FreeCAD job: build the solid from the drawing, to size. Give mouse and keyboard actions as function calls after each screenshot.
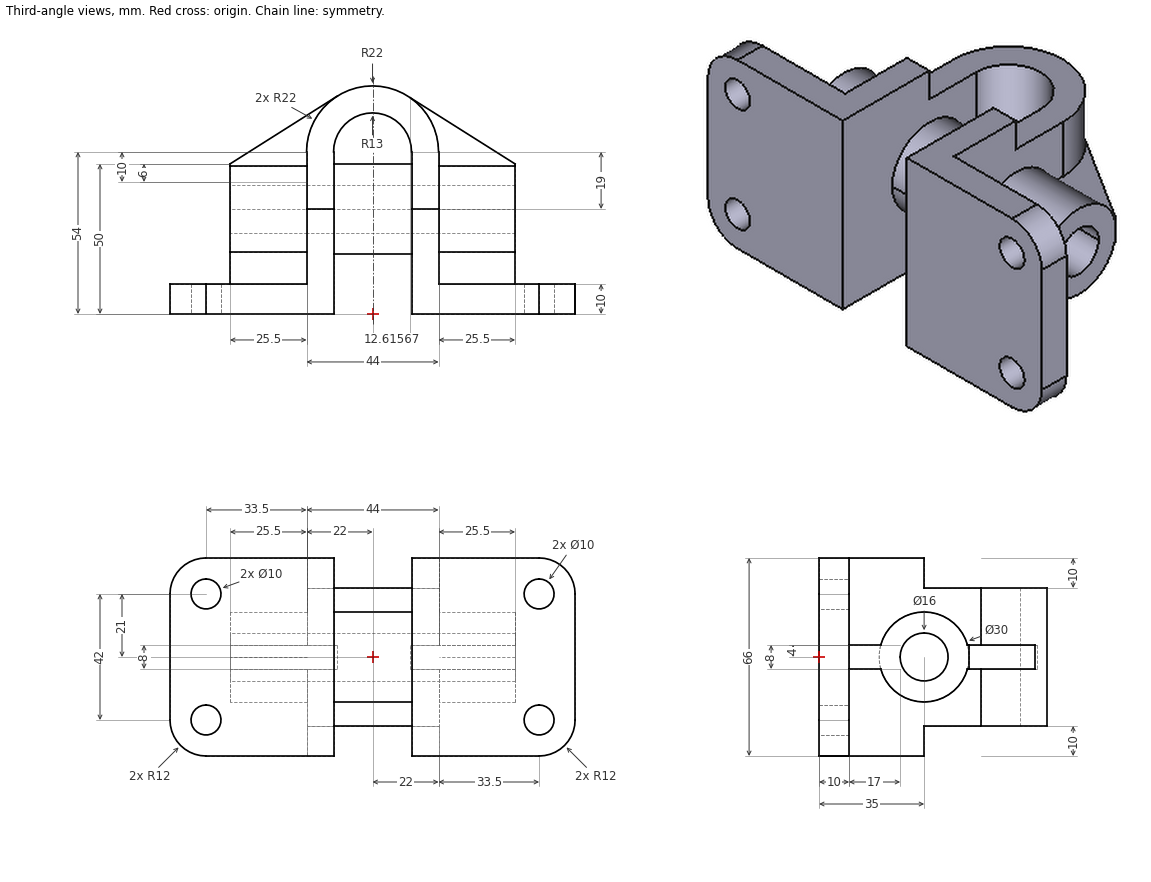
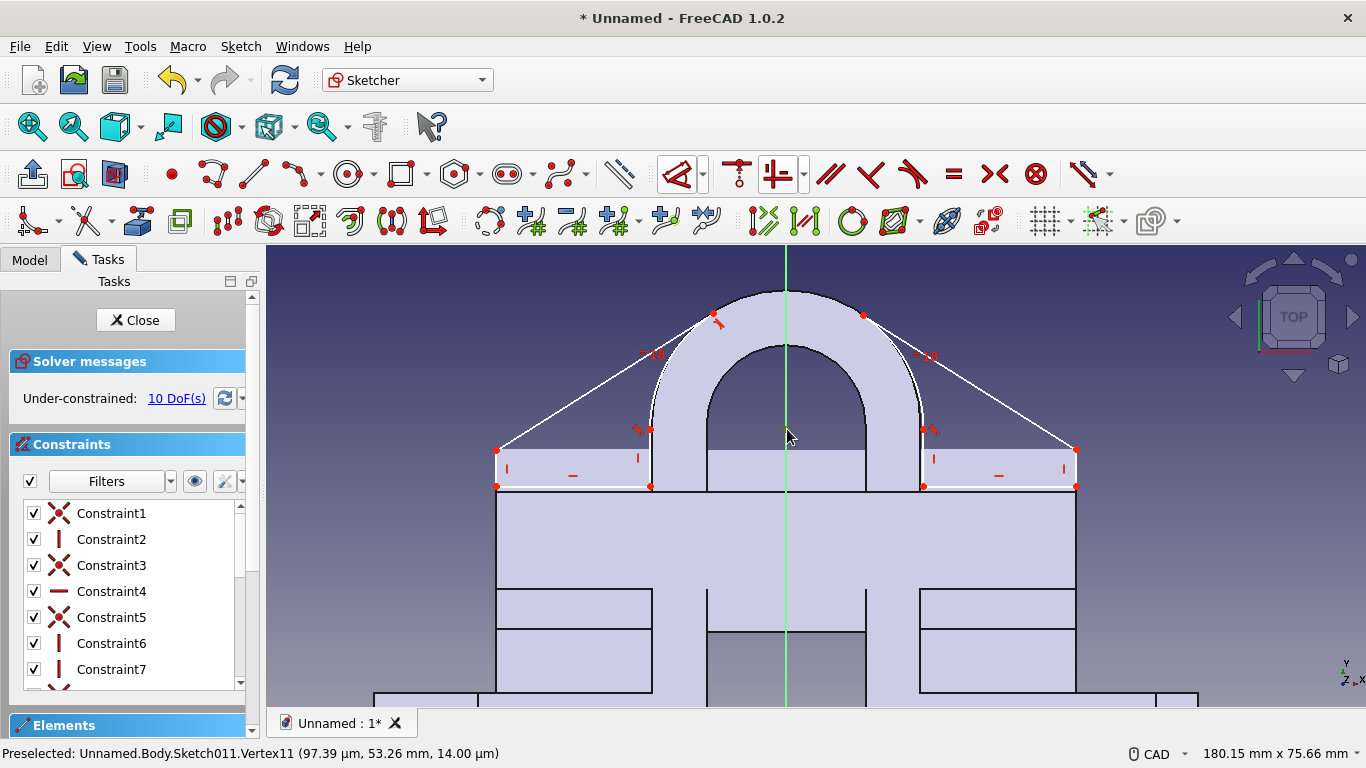
click(786, 650)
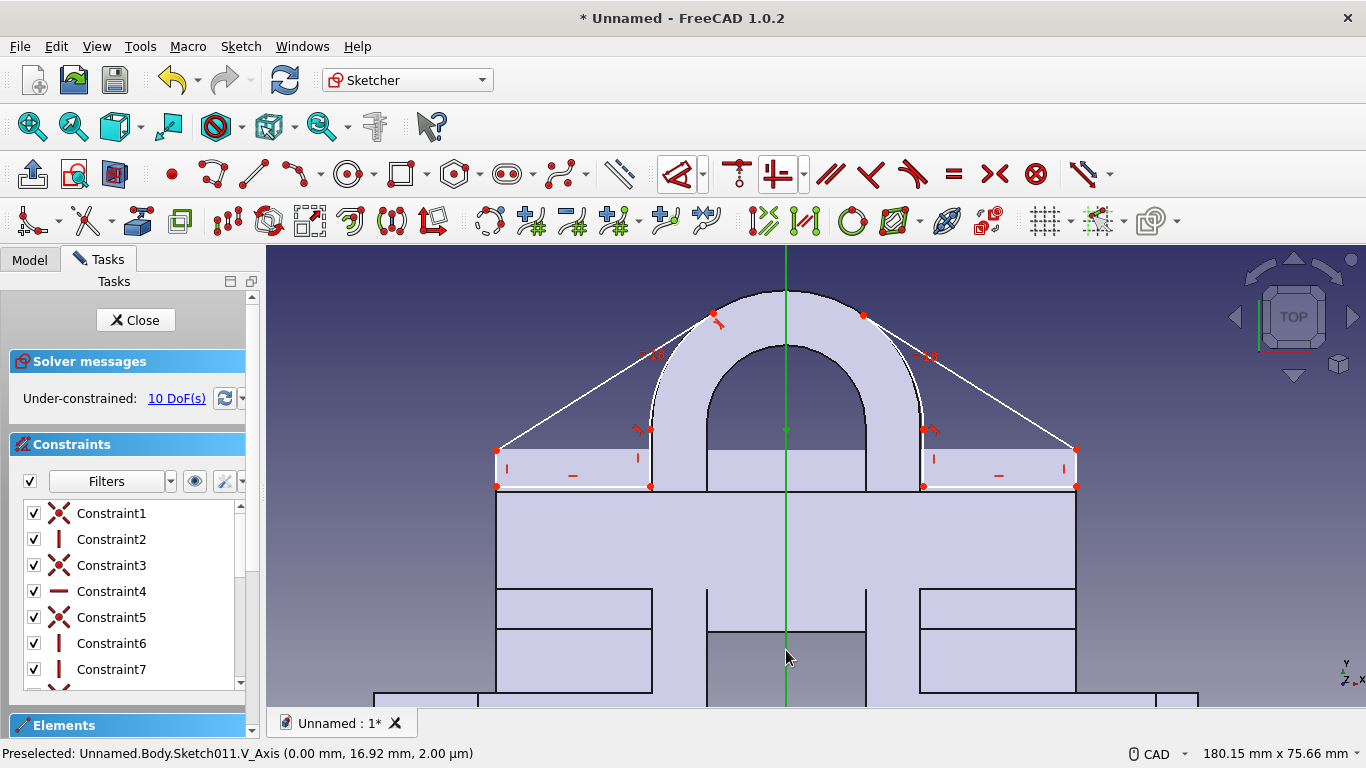
click(737, 174)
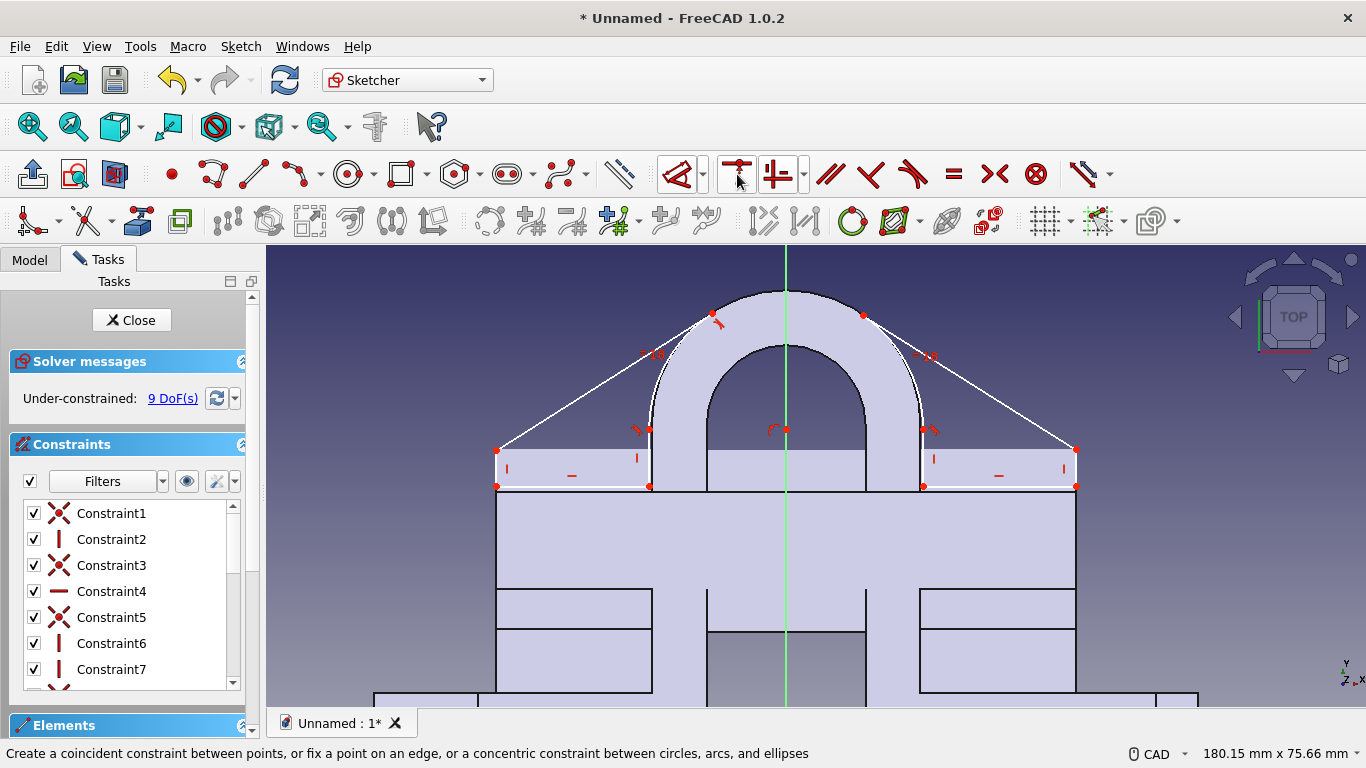
click(496, 487)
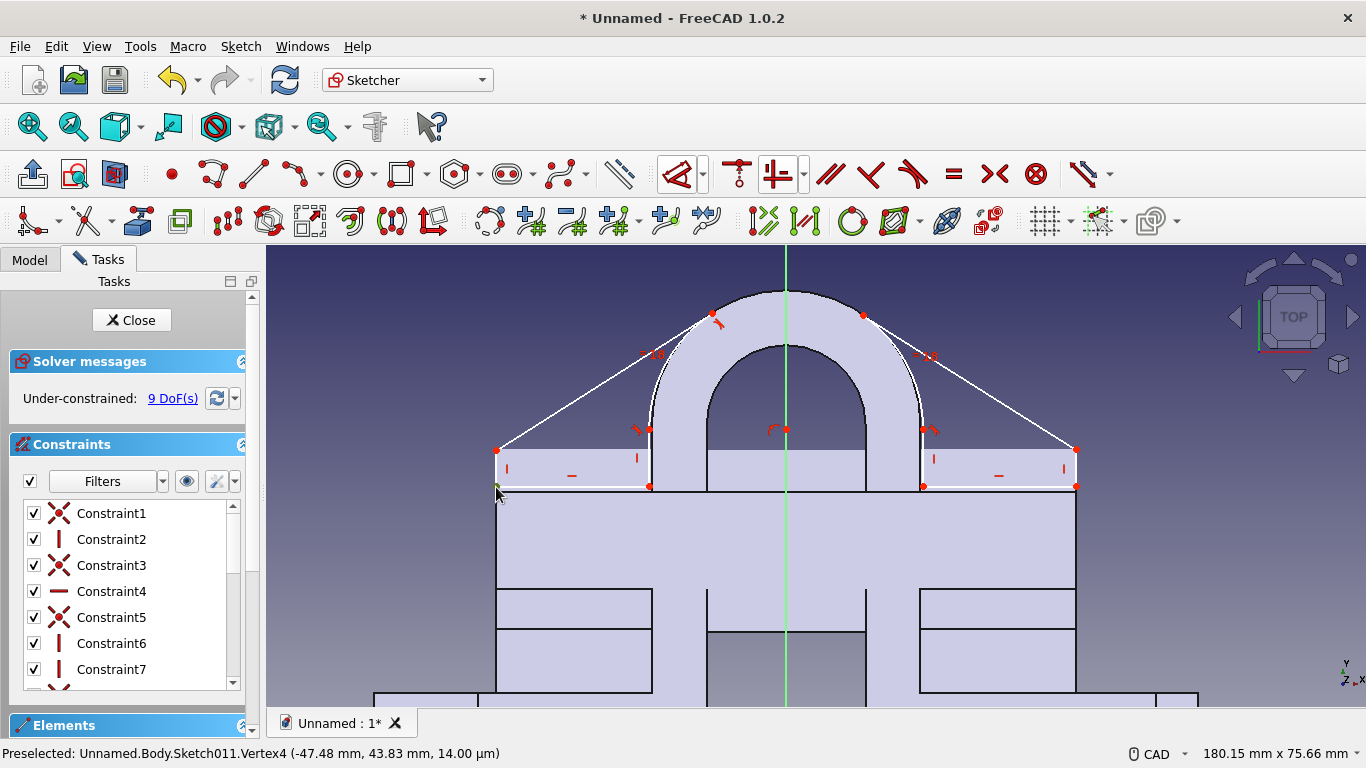
click(1076, 487)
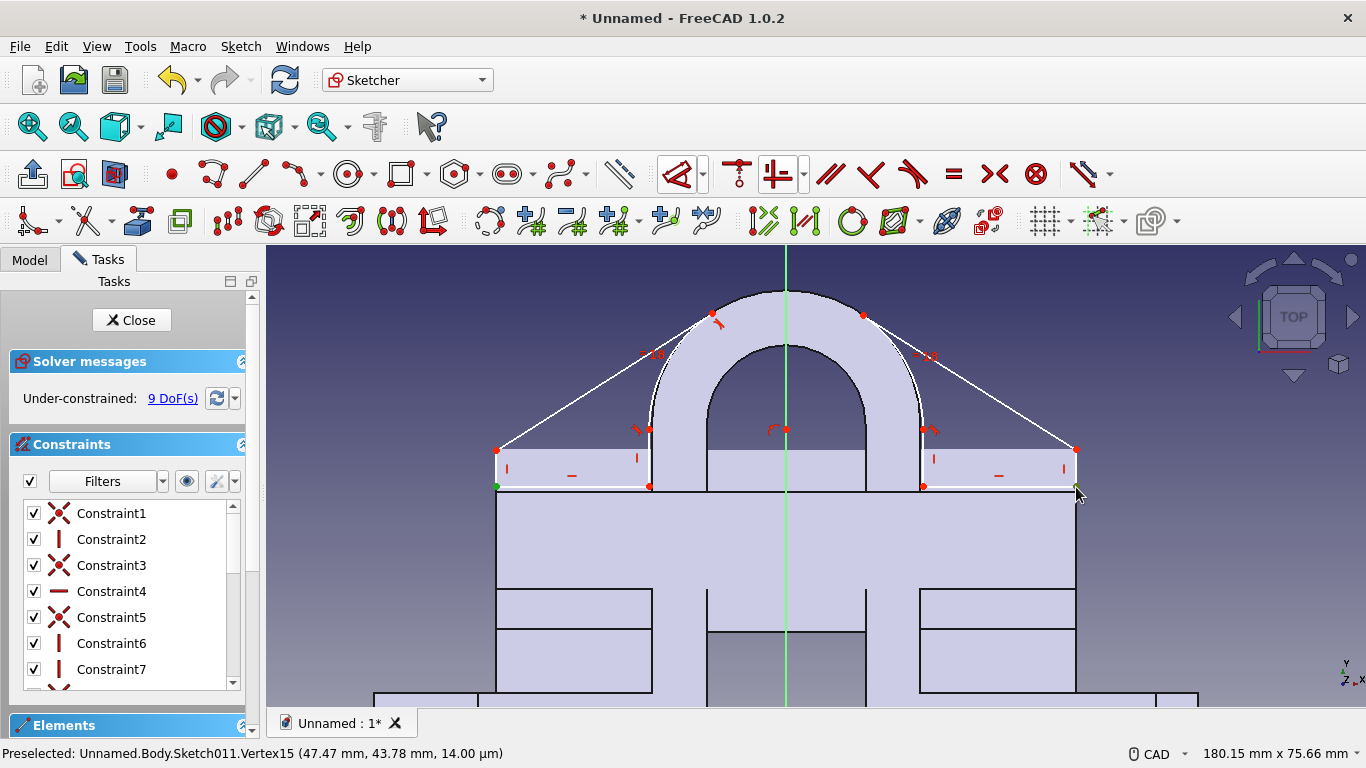
click(786, 650)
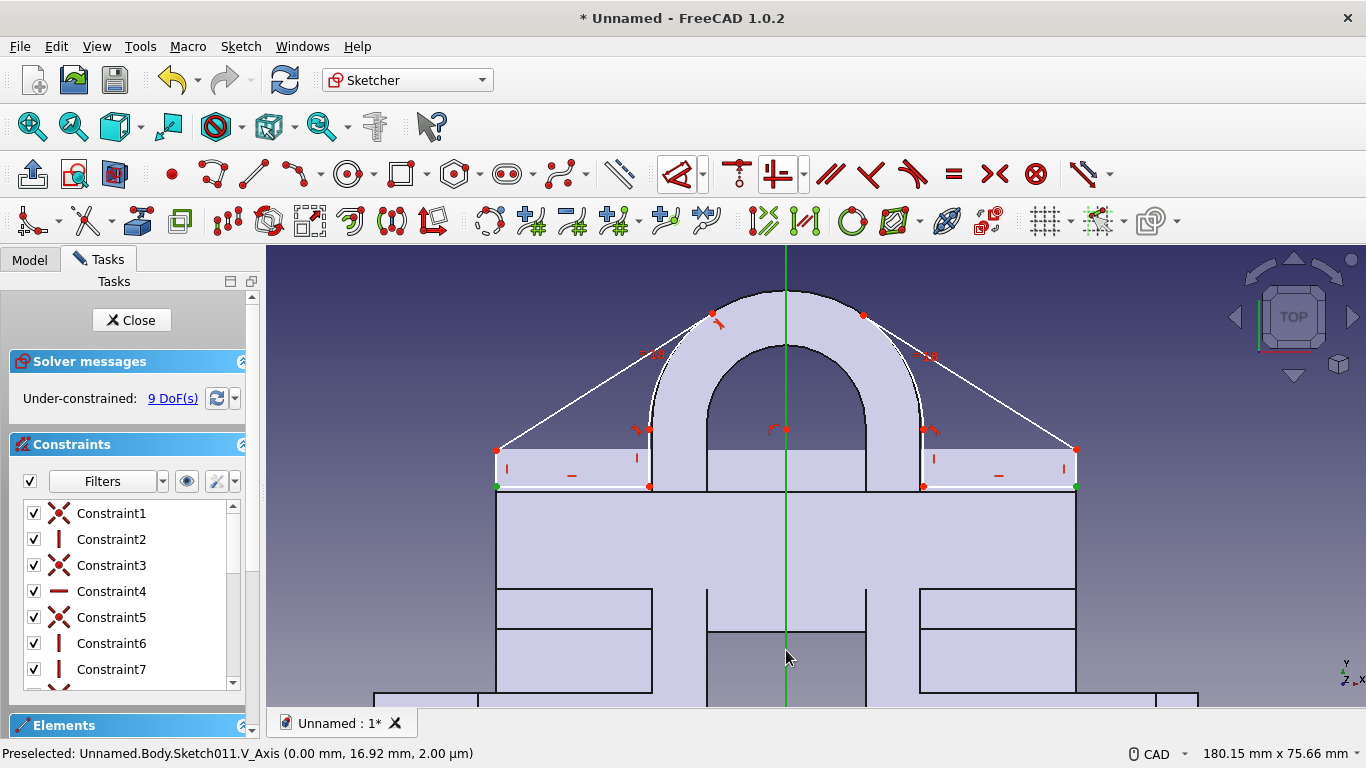
click(995, 174)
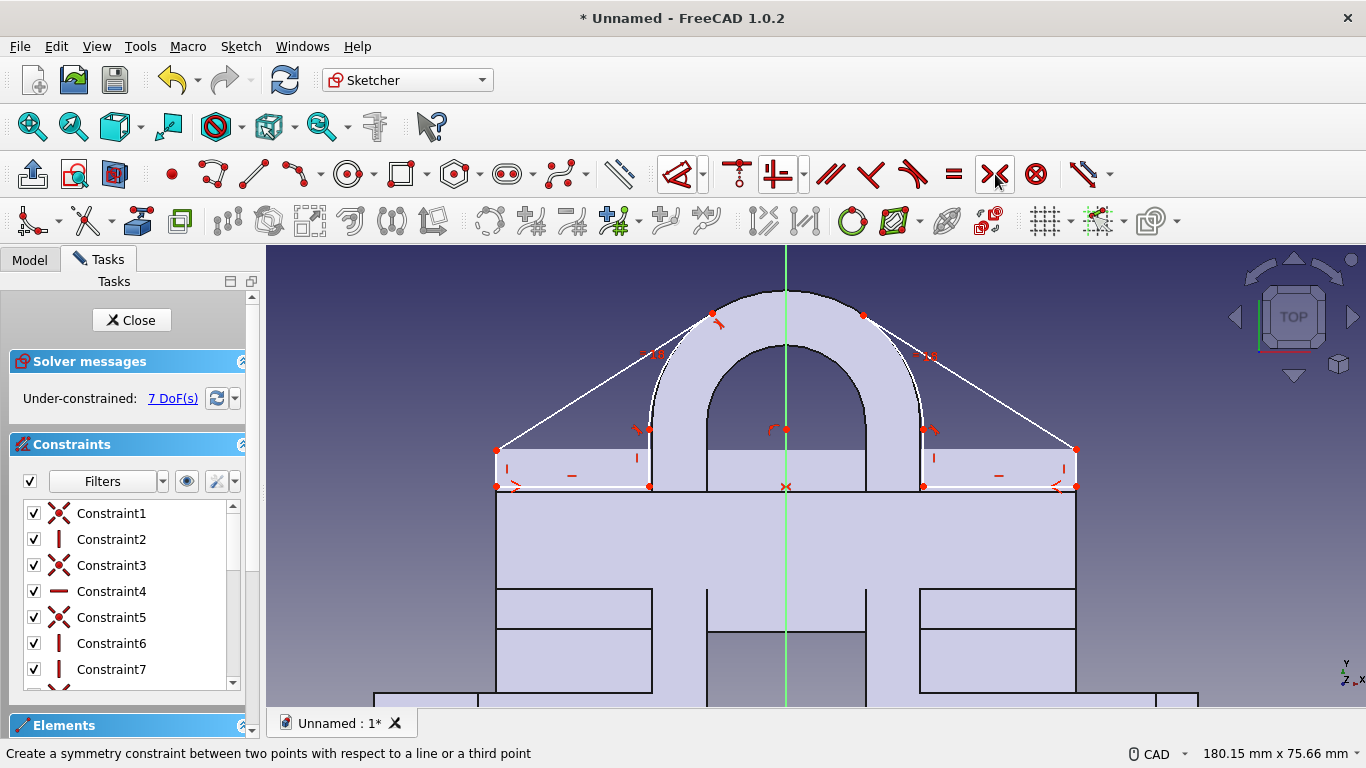
click(655, 388)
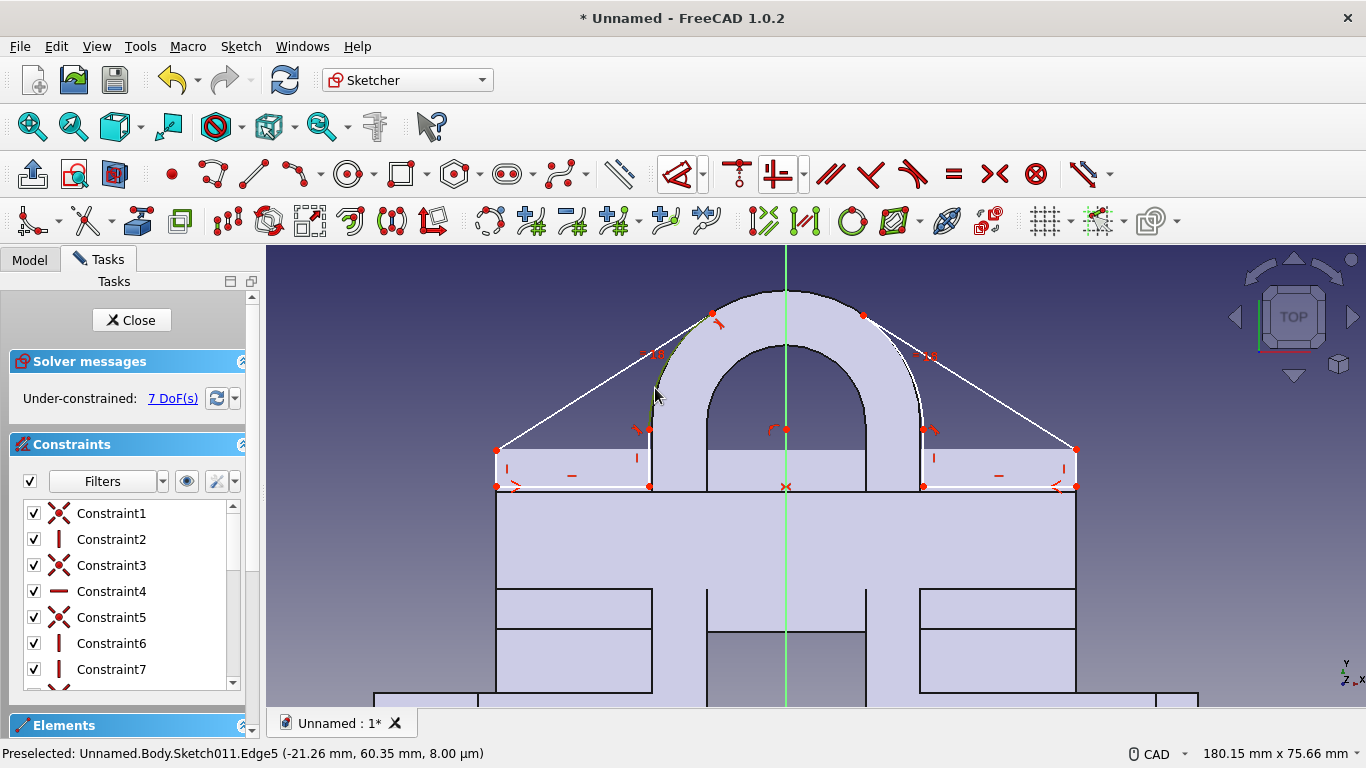
key(k)
key(r)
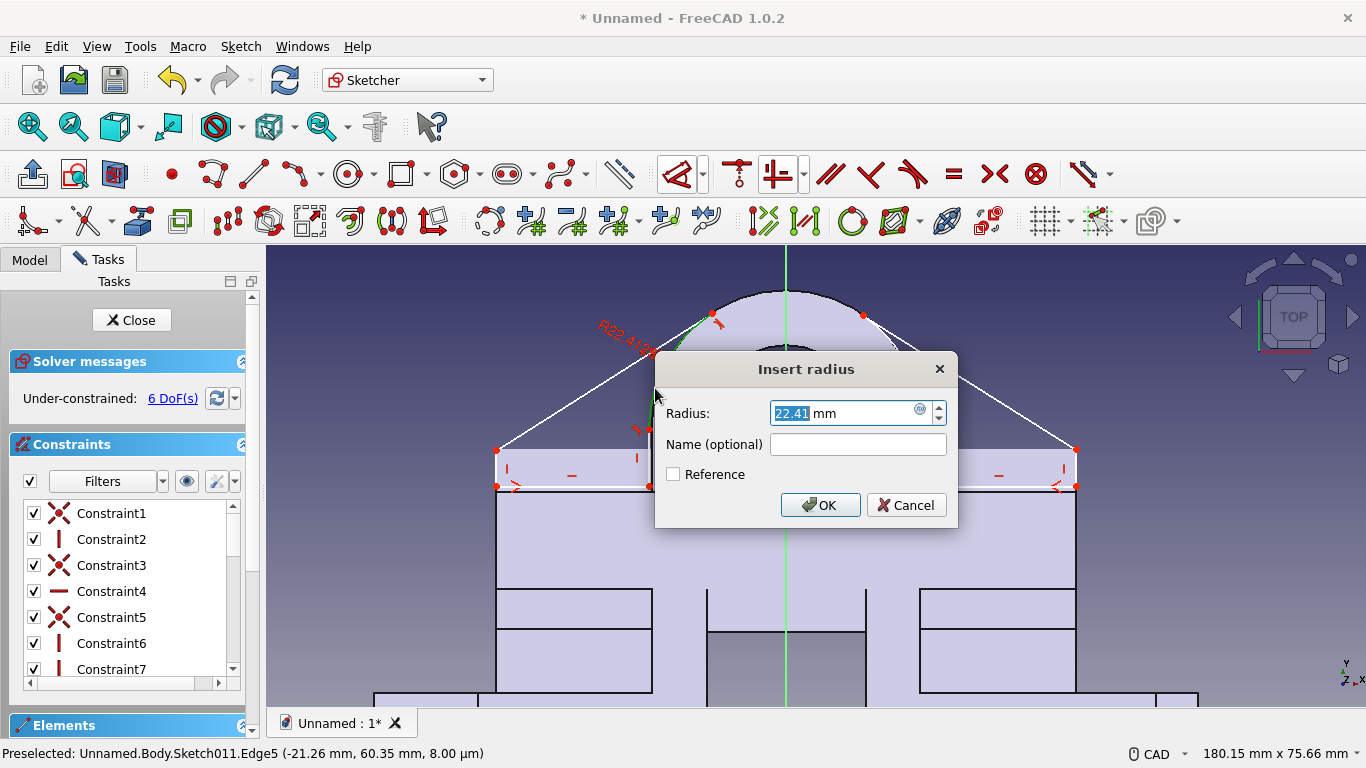
text(22)
key(Return)